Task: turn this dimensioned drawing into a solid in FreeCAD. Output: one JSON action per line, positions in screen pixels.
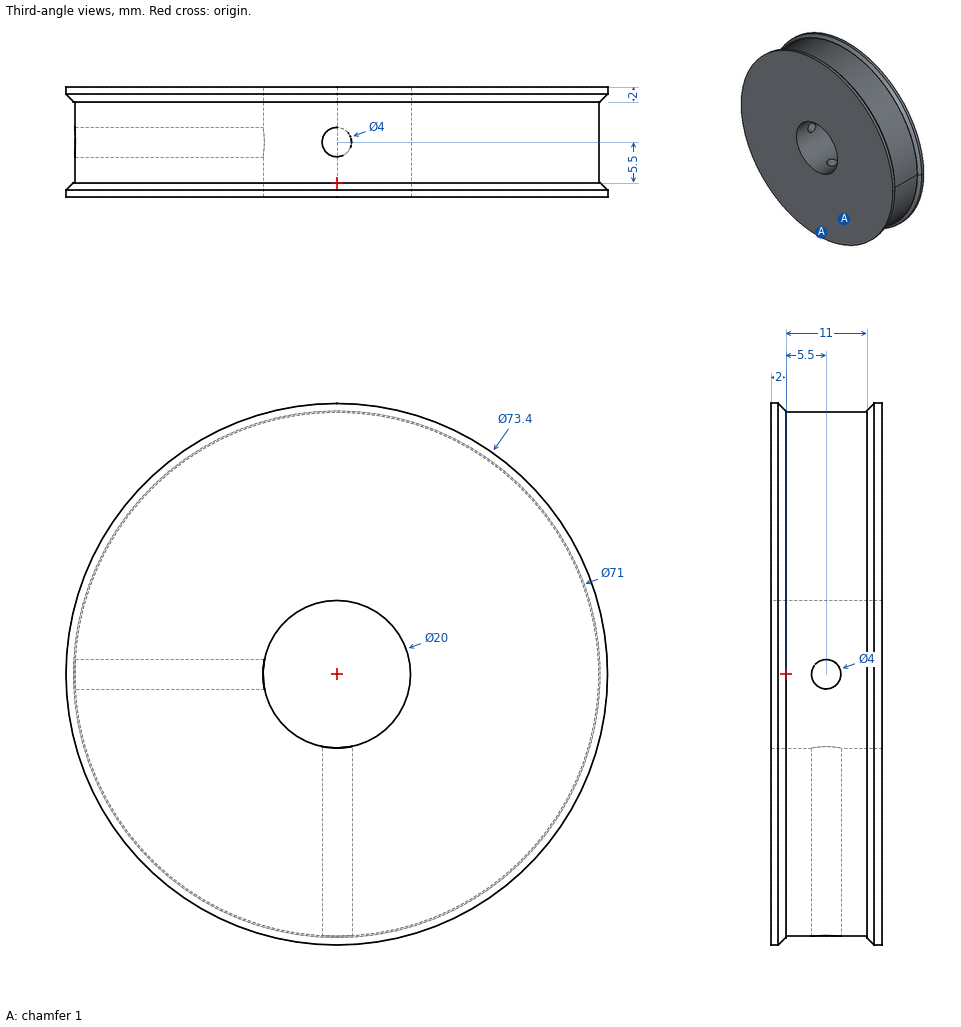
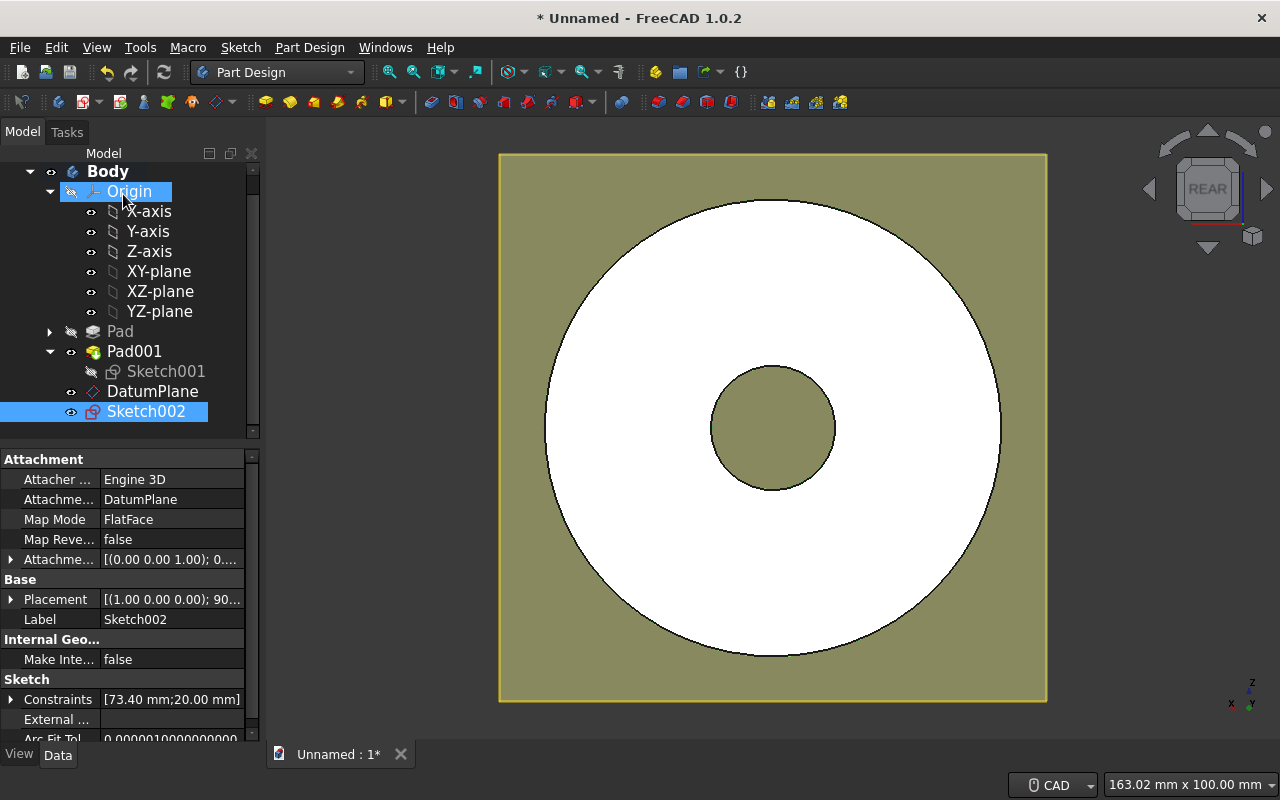
{"action": "left_click", "coordinate": [266, 102]}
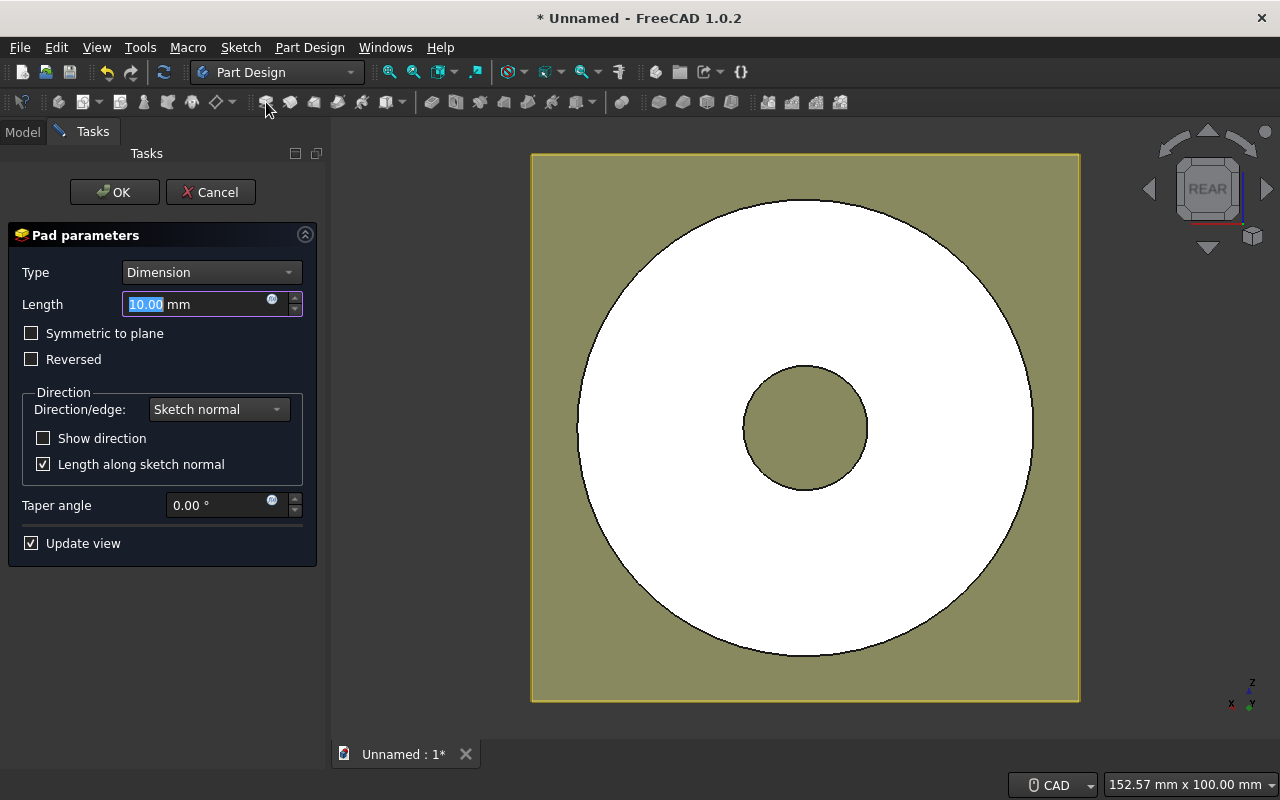
{"action": "type", "text": "2"}
{"action": "key", "text": "Tab"}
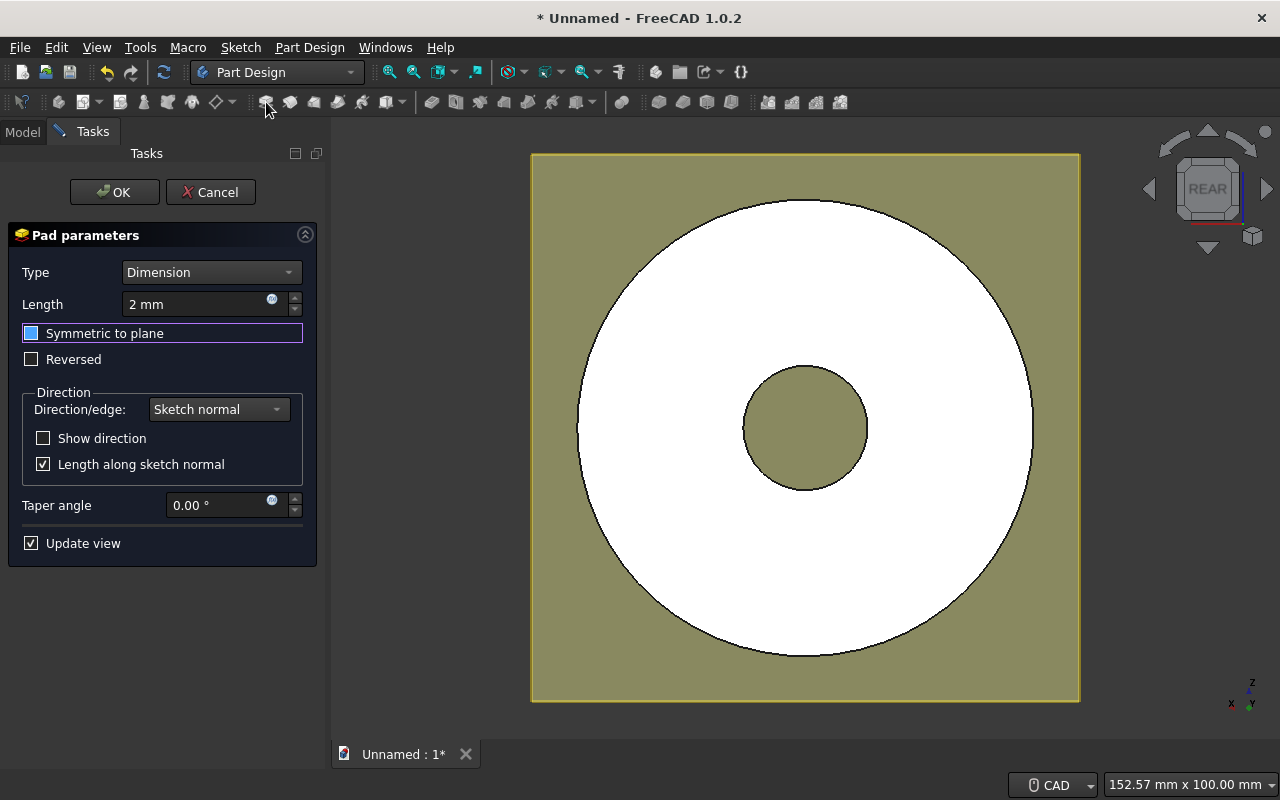
{"action": "left_click", "coordinate": [30, 359]}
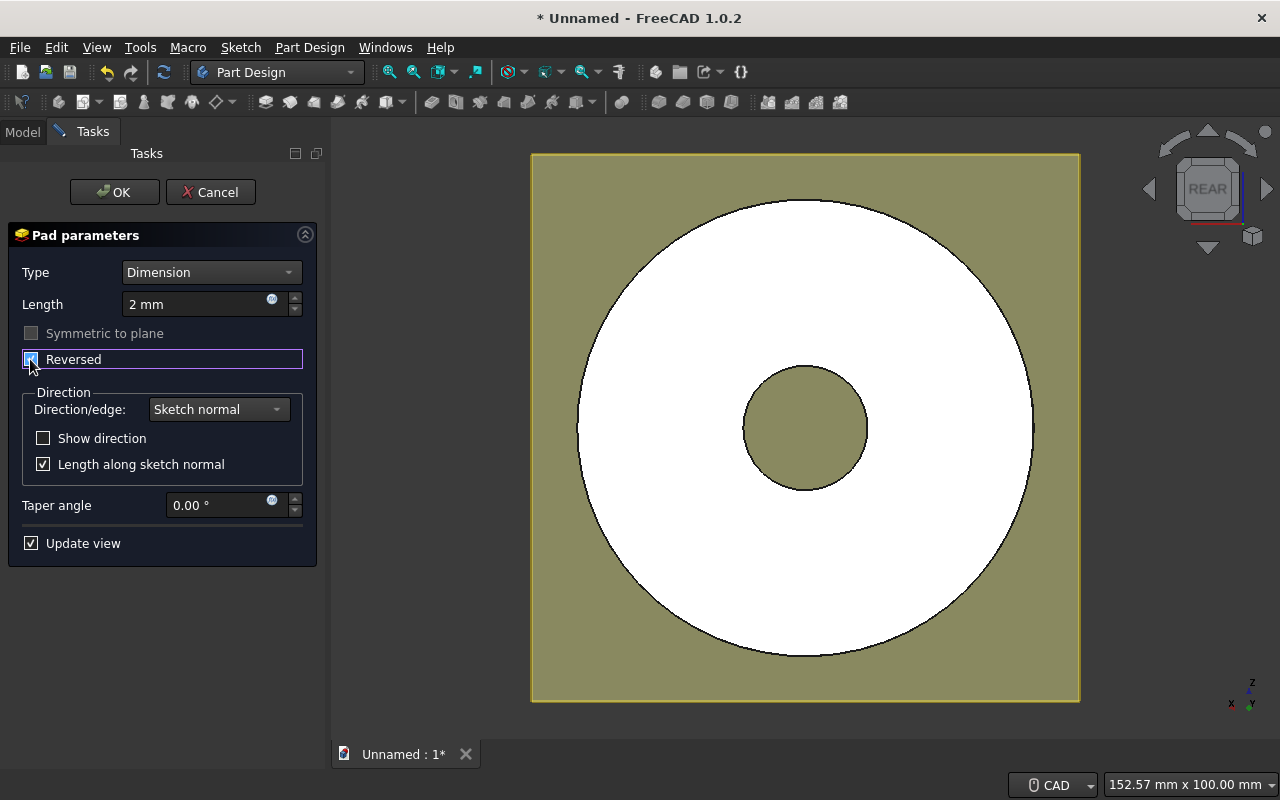
{"action": "left_click", "coordinate": [115, 192]}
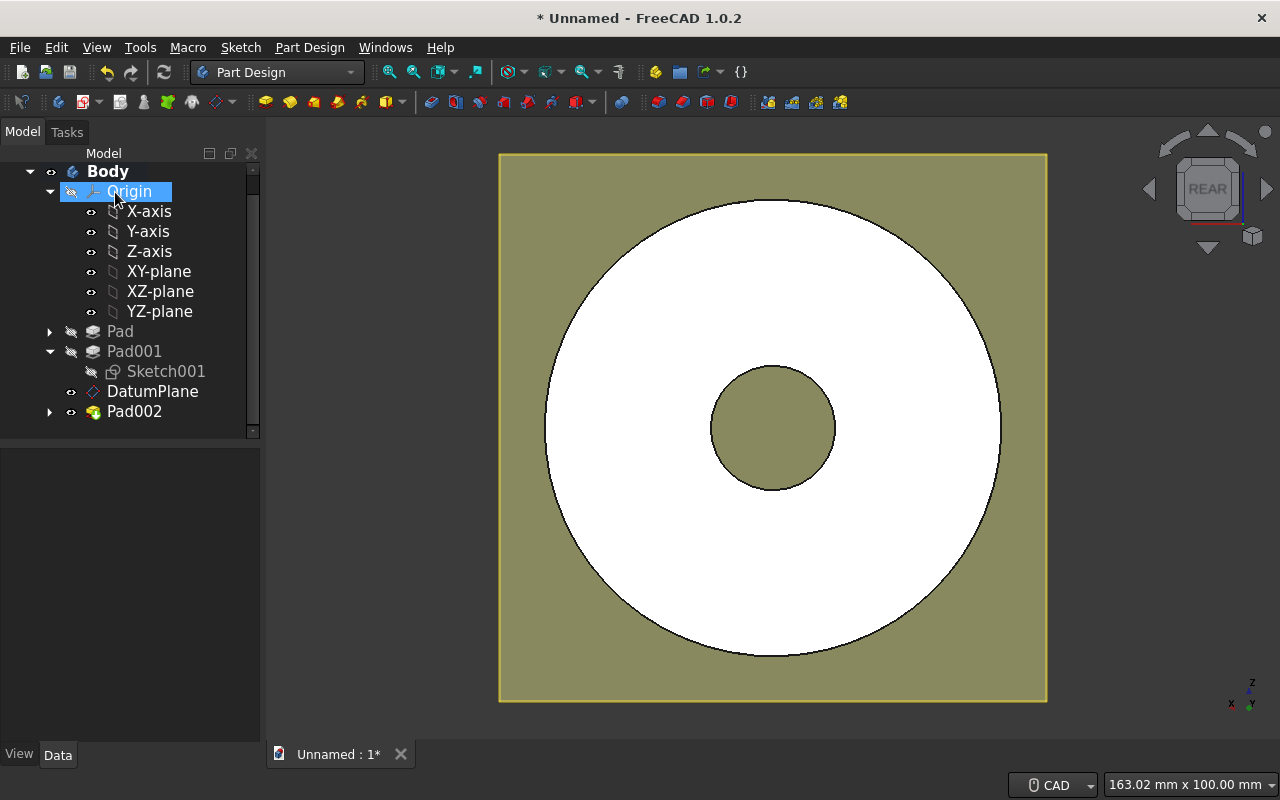
{"action": "left_click", "coordinate": [116, 392]}
{"action": "key", "text": "space"}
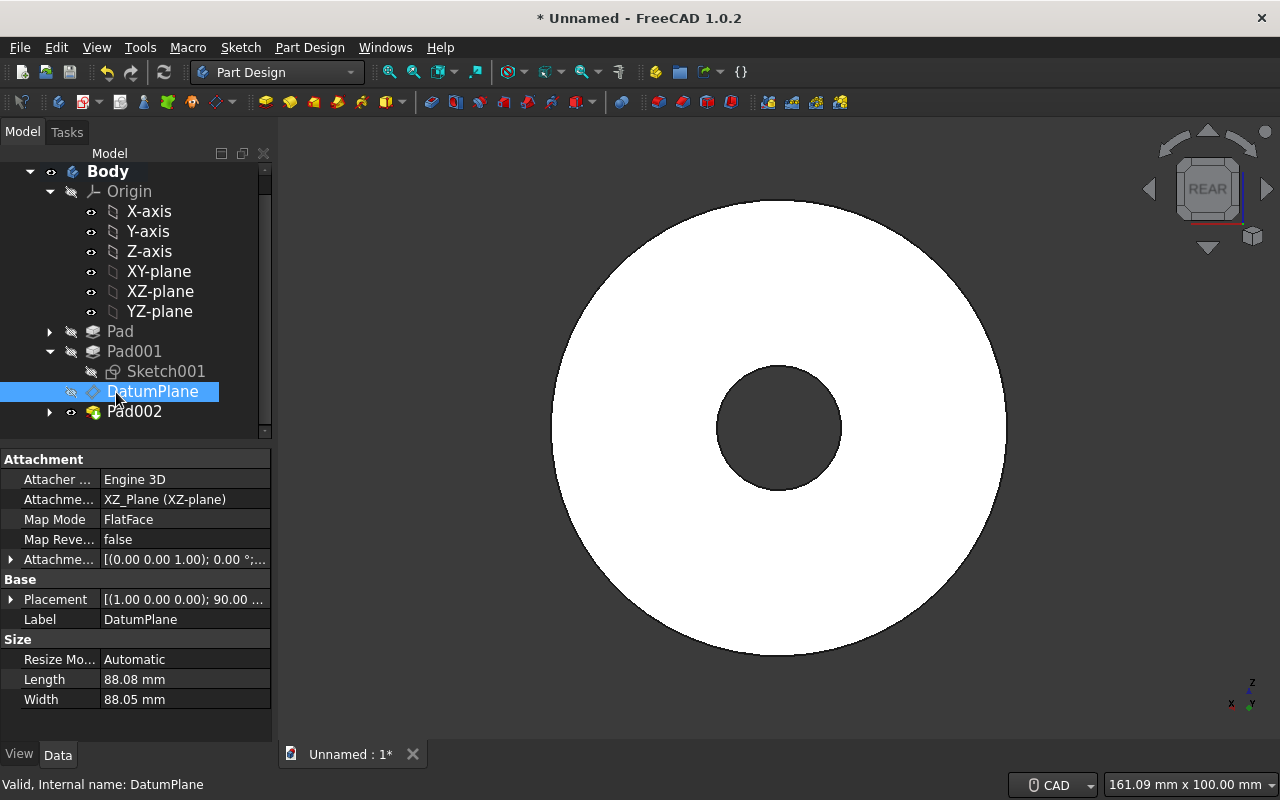
{"action": "key", "text": "0"}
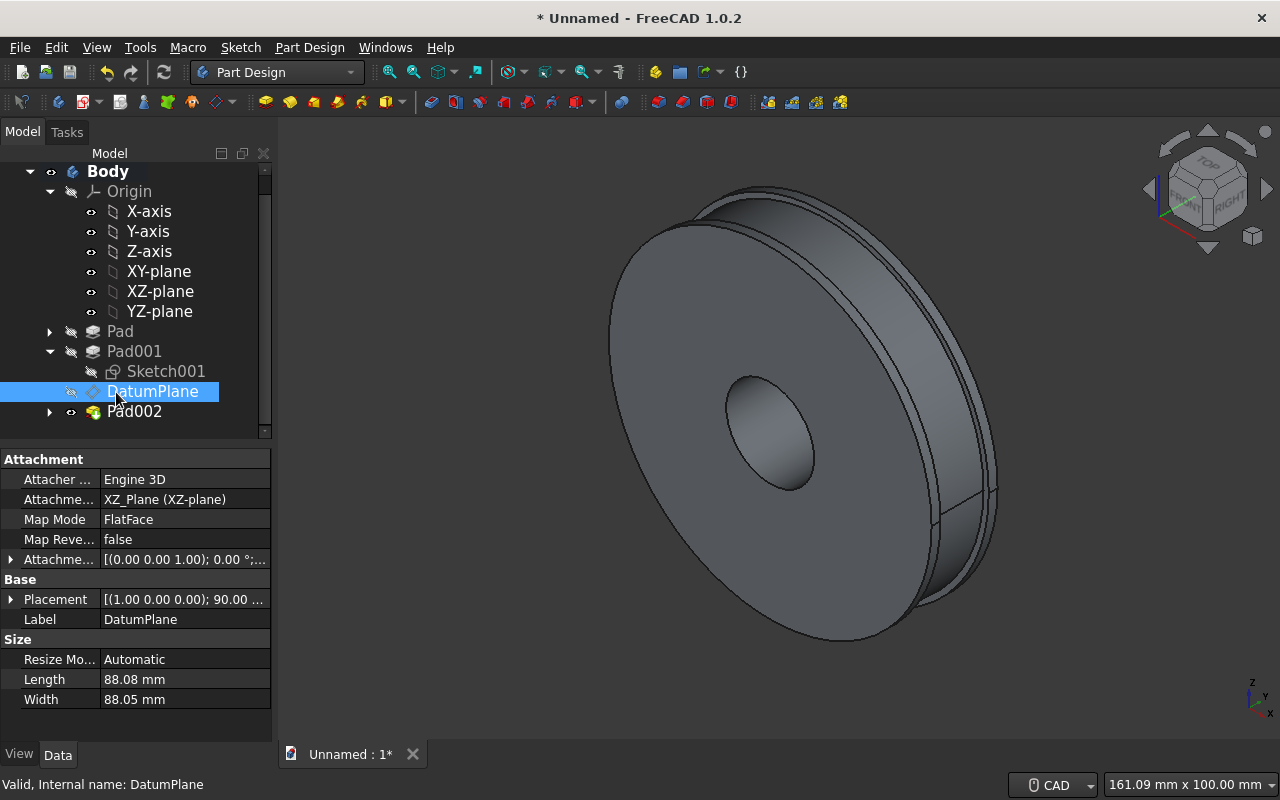
{"action": "left_click", "coordinate": [390, 72]}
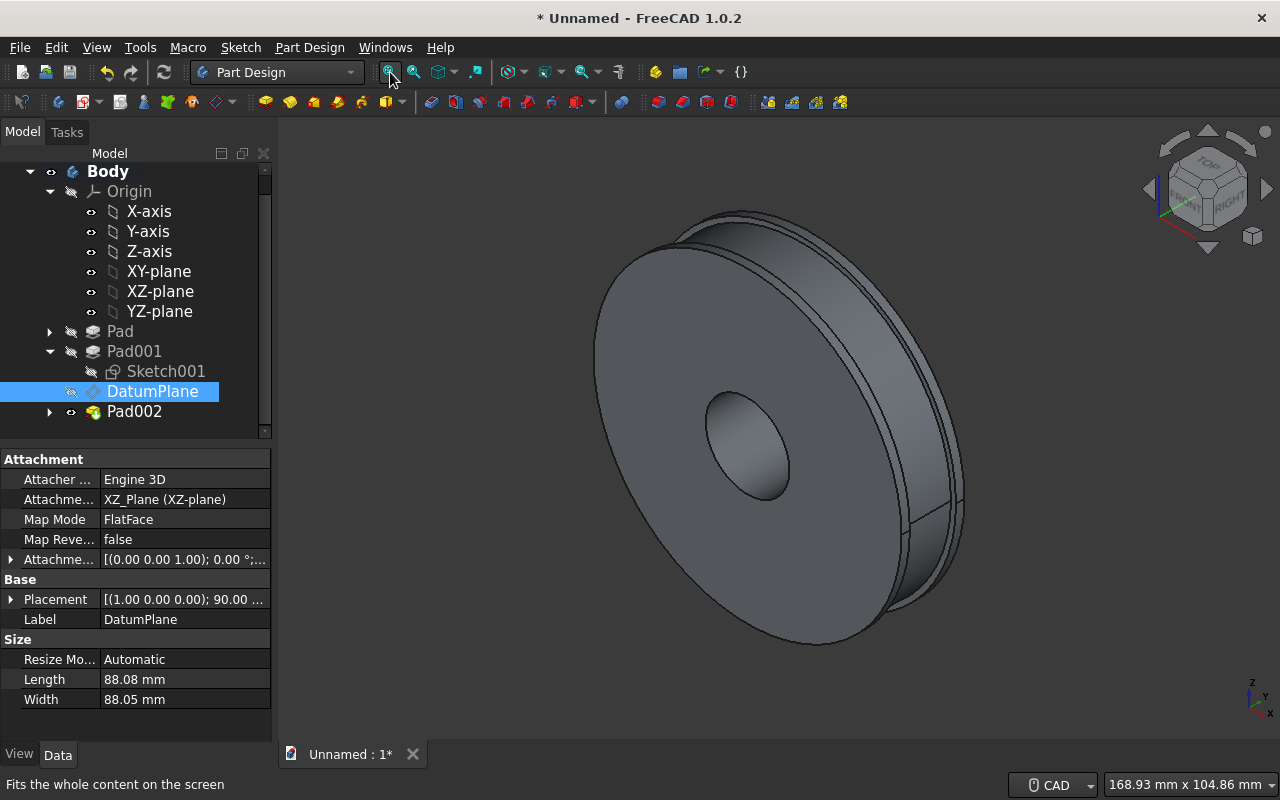
{"action": "left_click", "coordinate": [755, 217]}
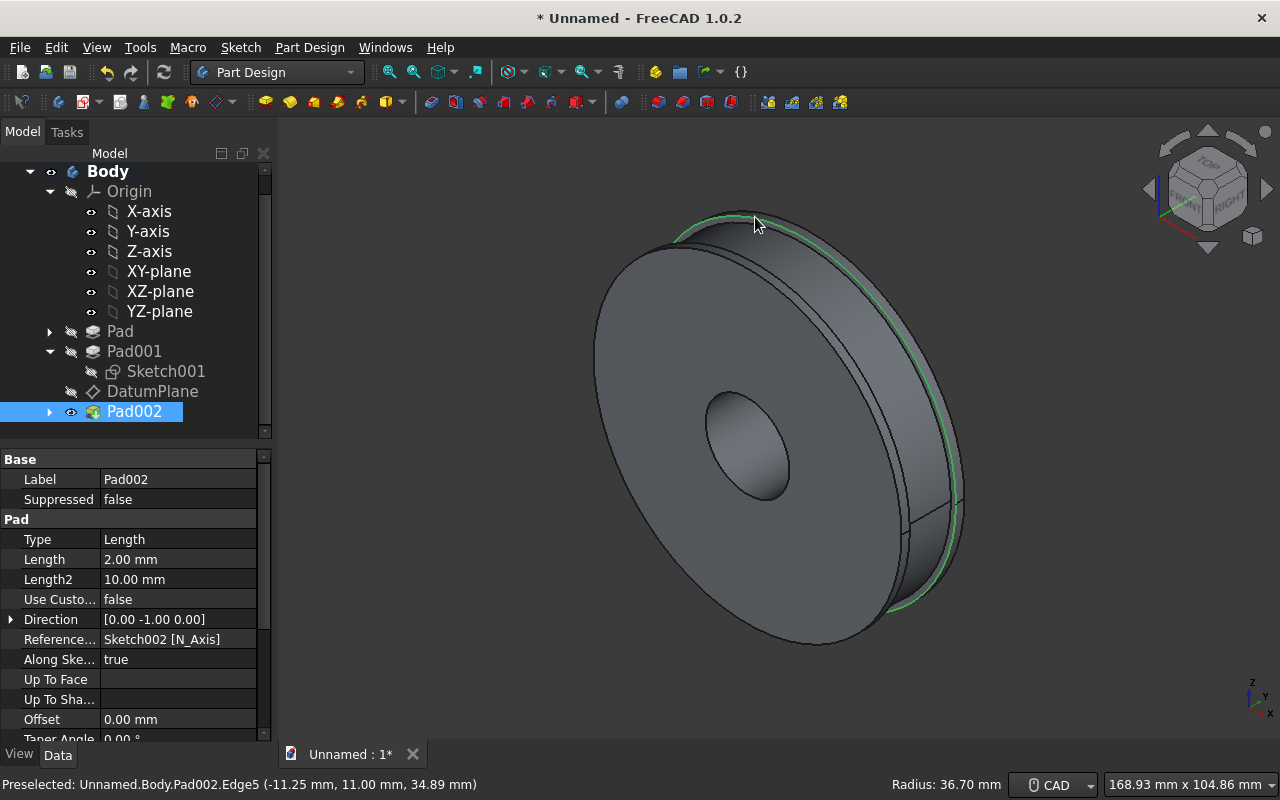
{"action": "key", "text": "2"}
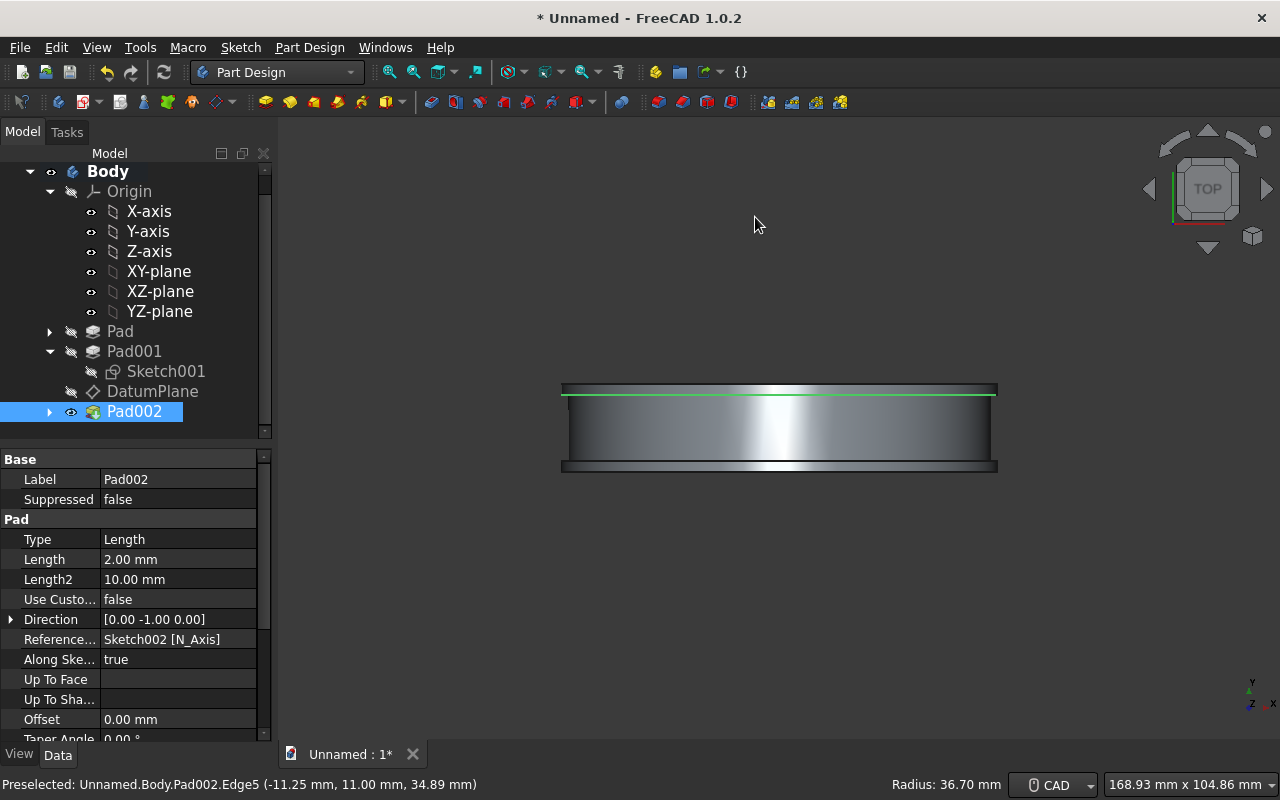
{"action": "left_click", "coordinate": [390, 72]}